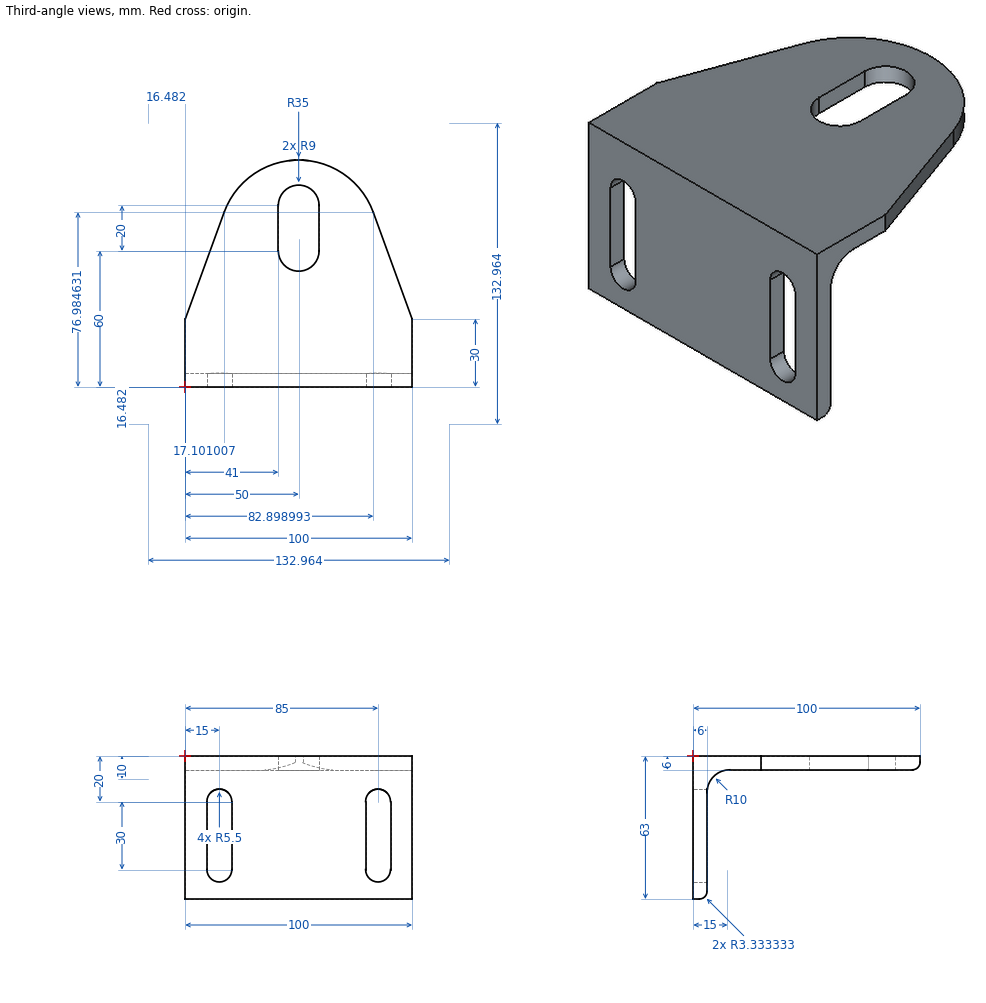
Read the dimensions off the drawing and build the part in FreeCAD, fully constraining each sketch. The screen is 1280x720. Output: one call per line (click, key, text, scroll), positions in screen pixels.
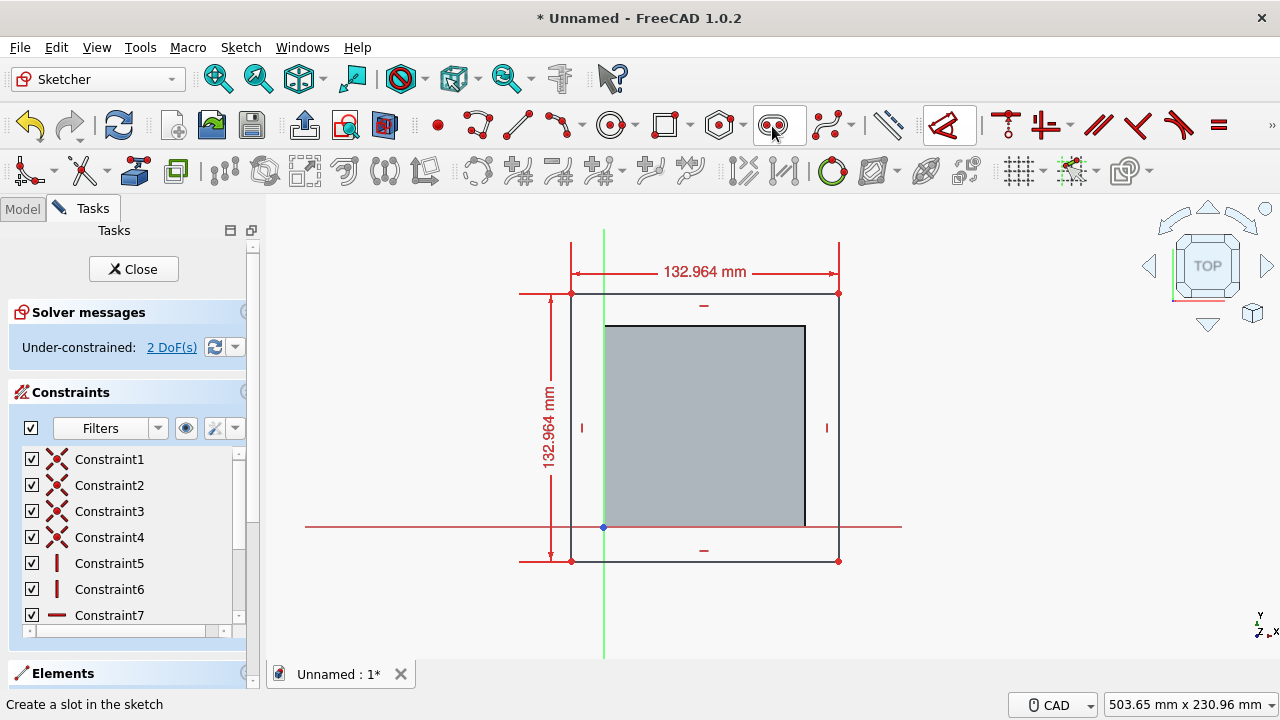
scroll(705, 407, up, 2)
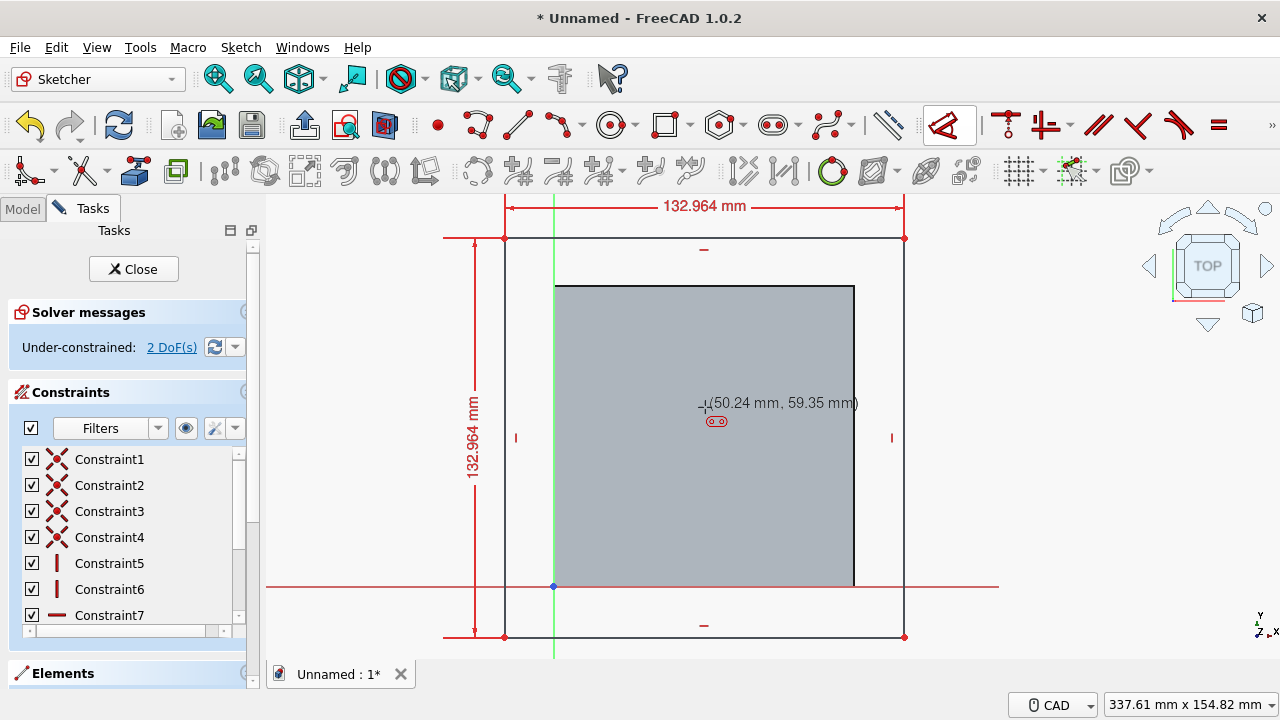
click(704, 406)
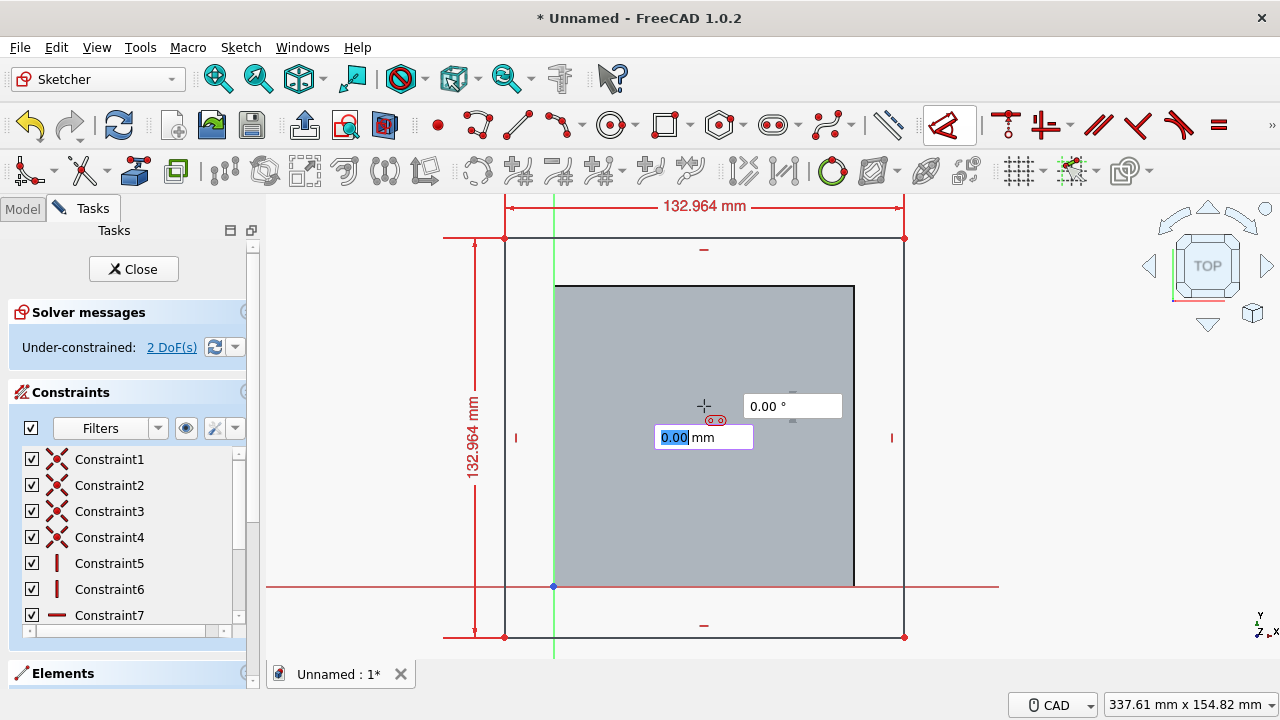
click(704, 346)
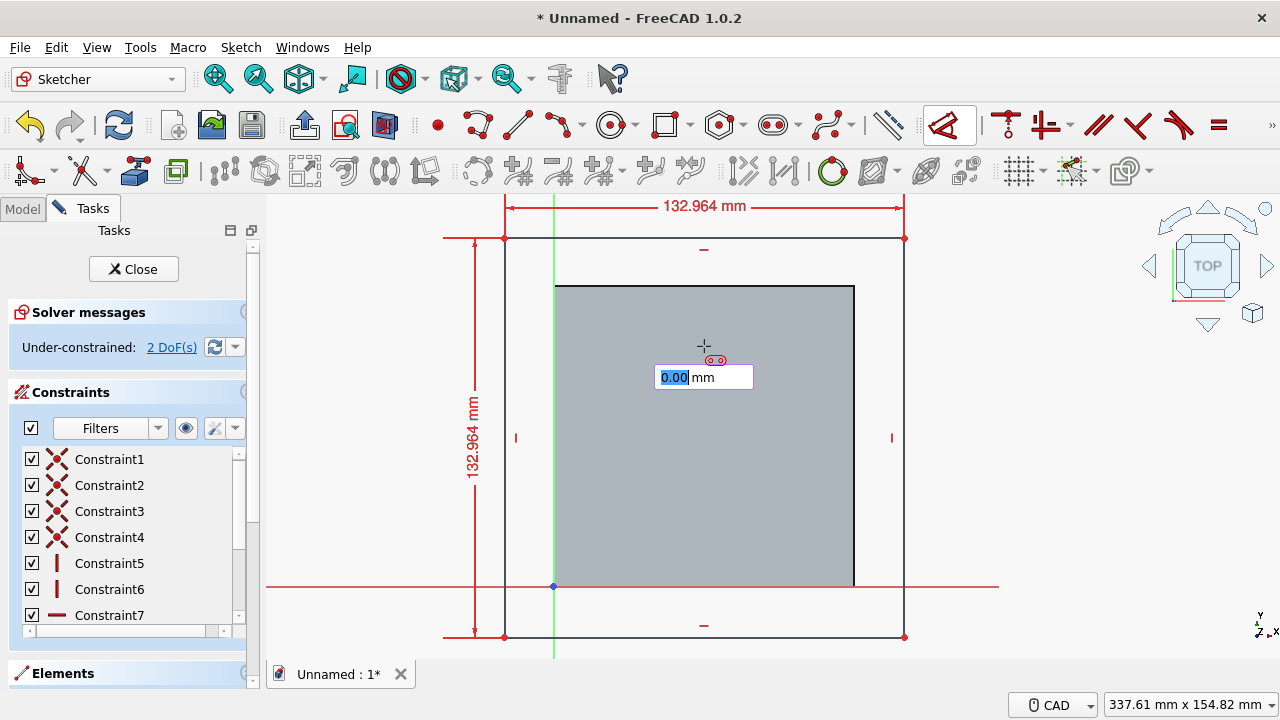
click(731, 376)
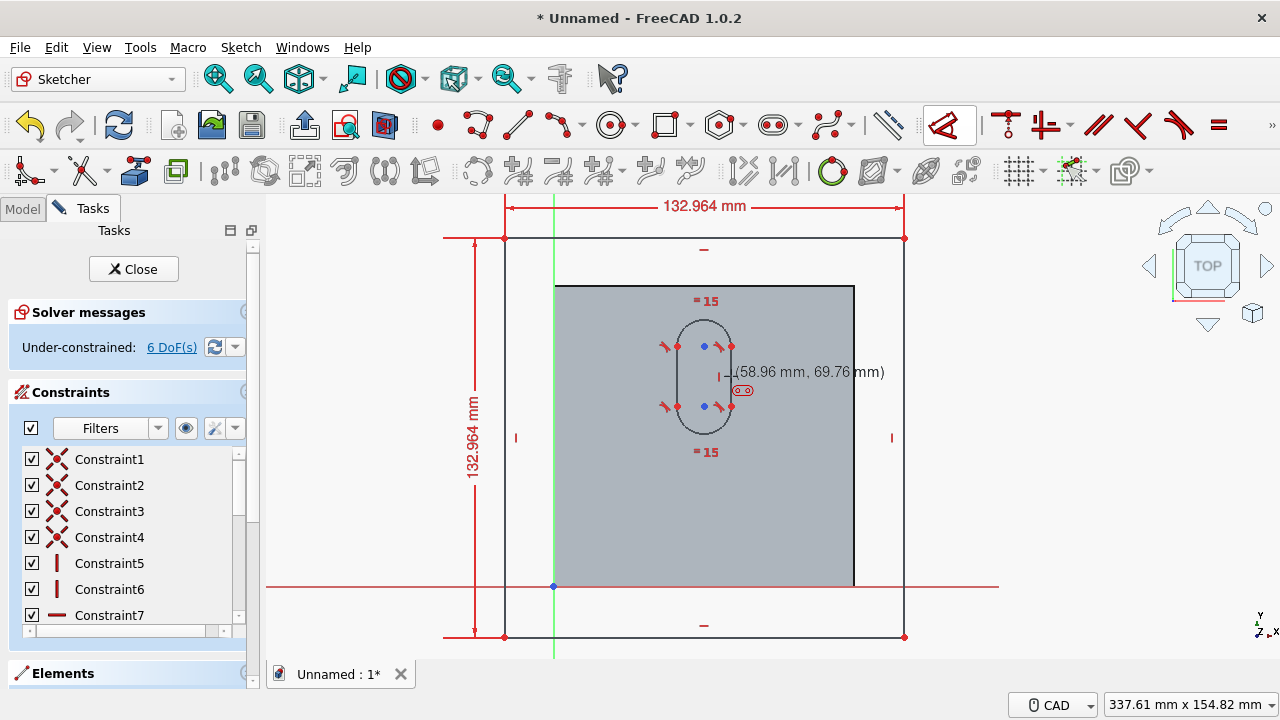
click(478, 126)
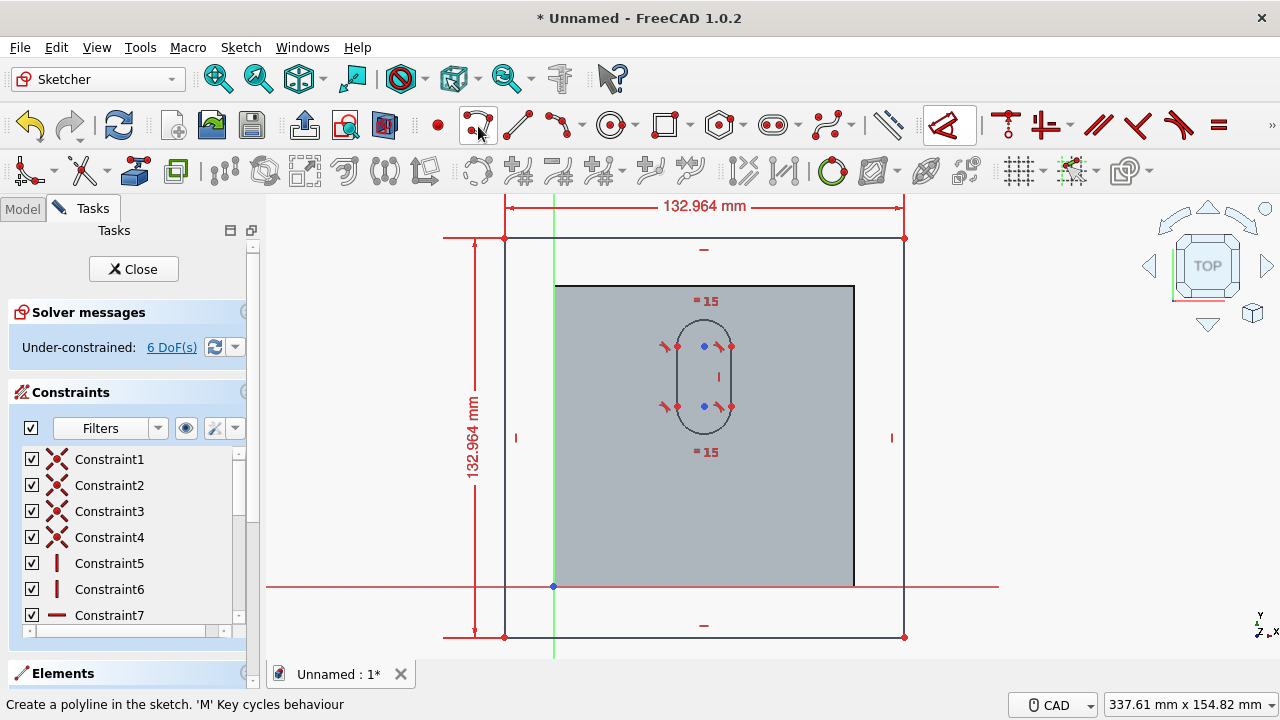
click(803, 355)
click(854, 496)
click(854, 587)
click(554, 587)
click(563, 496)
click(605, 355)
right_click(605, 355)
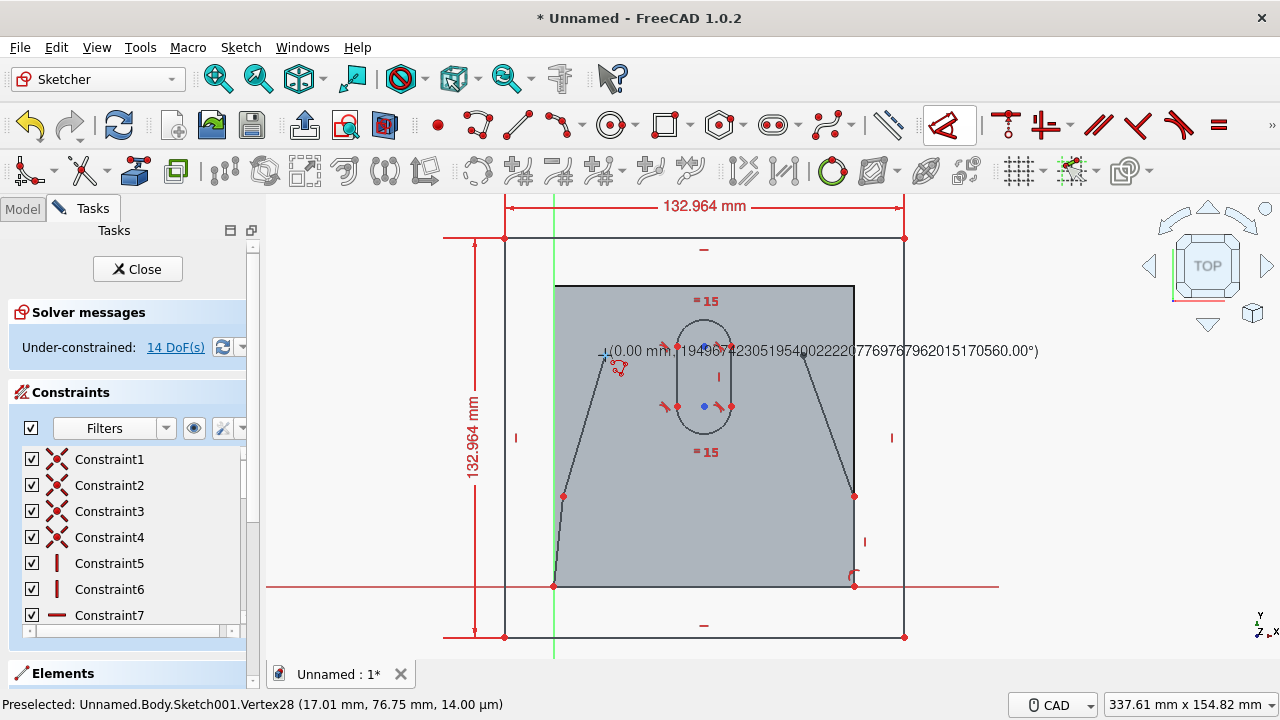
click(558, 126)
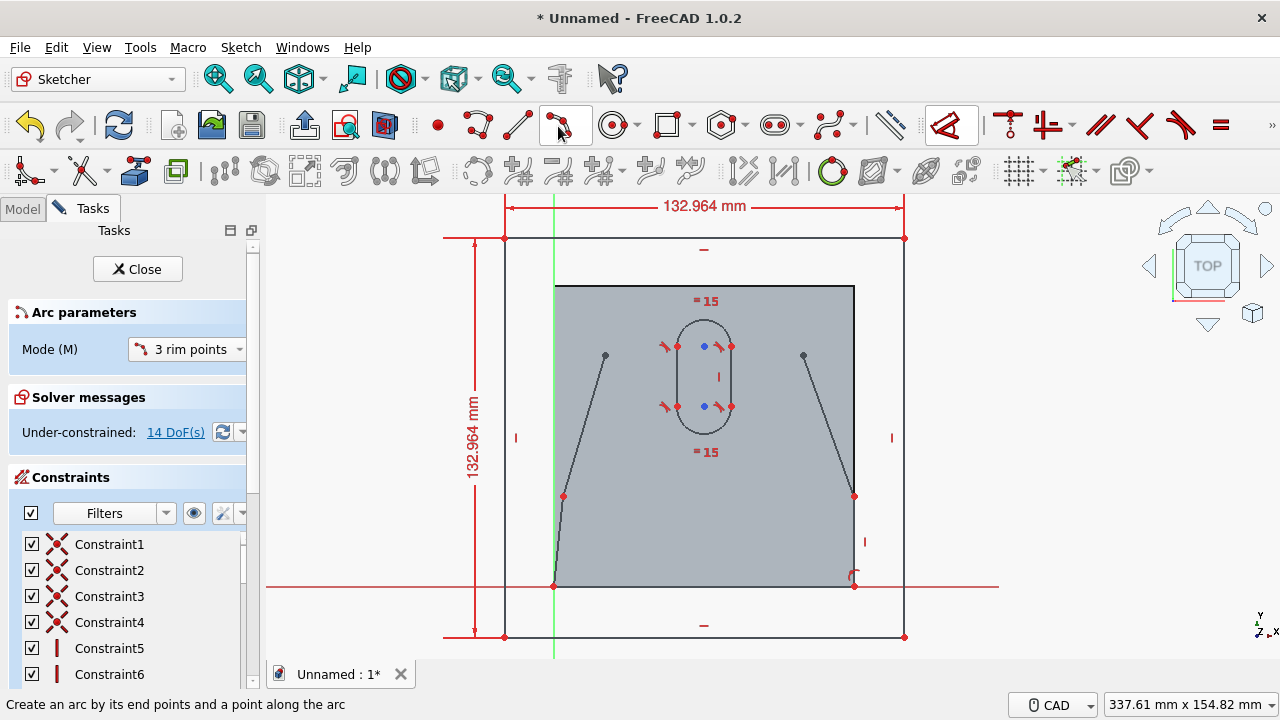
click(605, 356)
click(803, 356)
click(704, 286)
key(Escape)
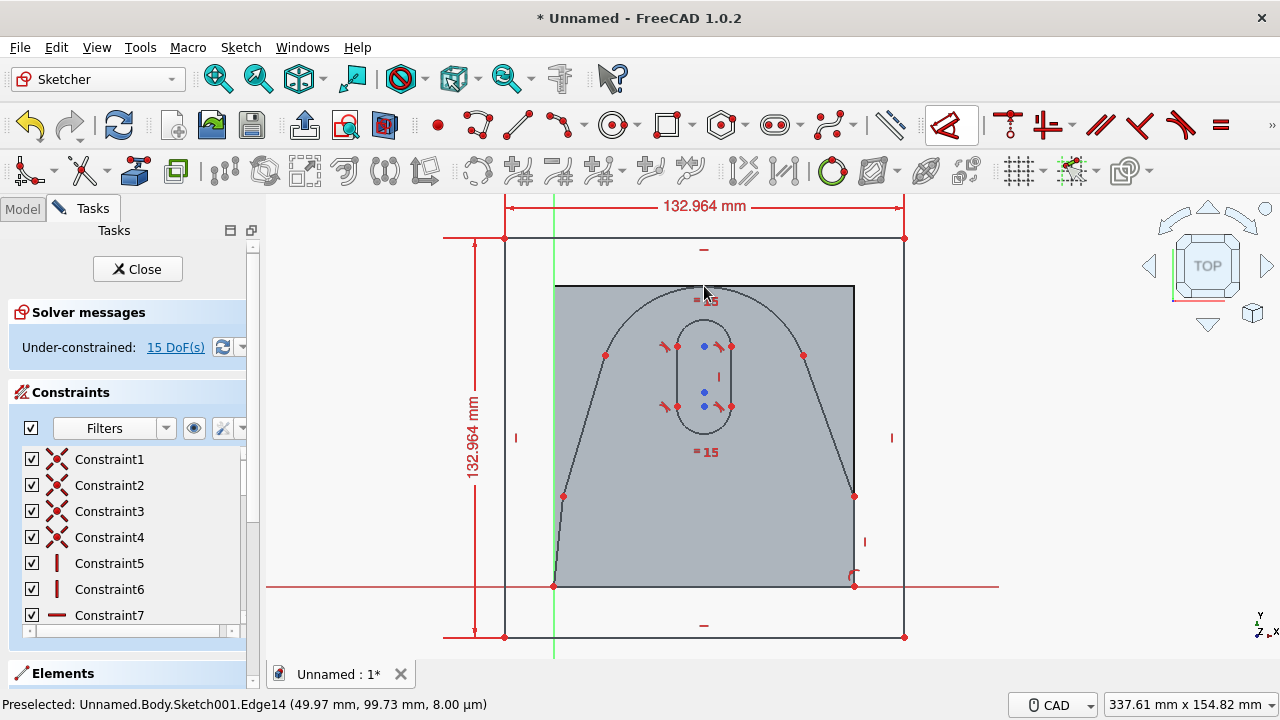
click(557, 560)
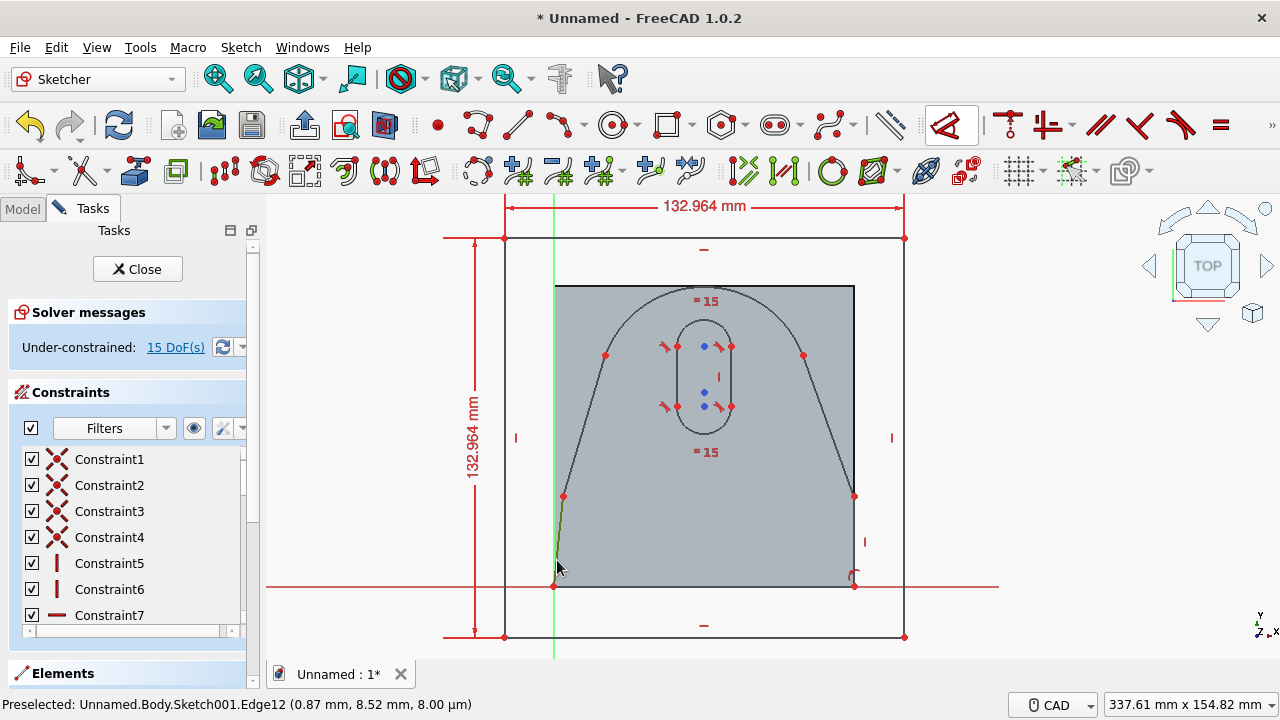
key(v)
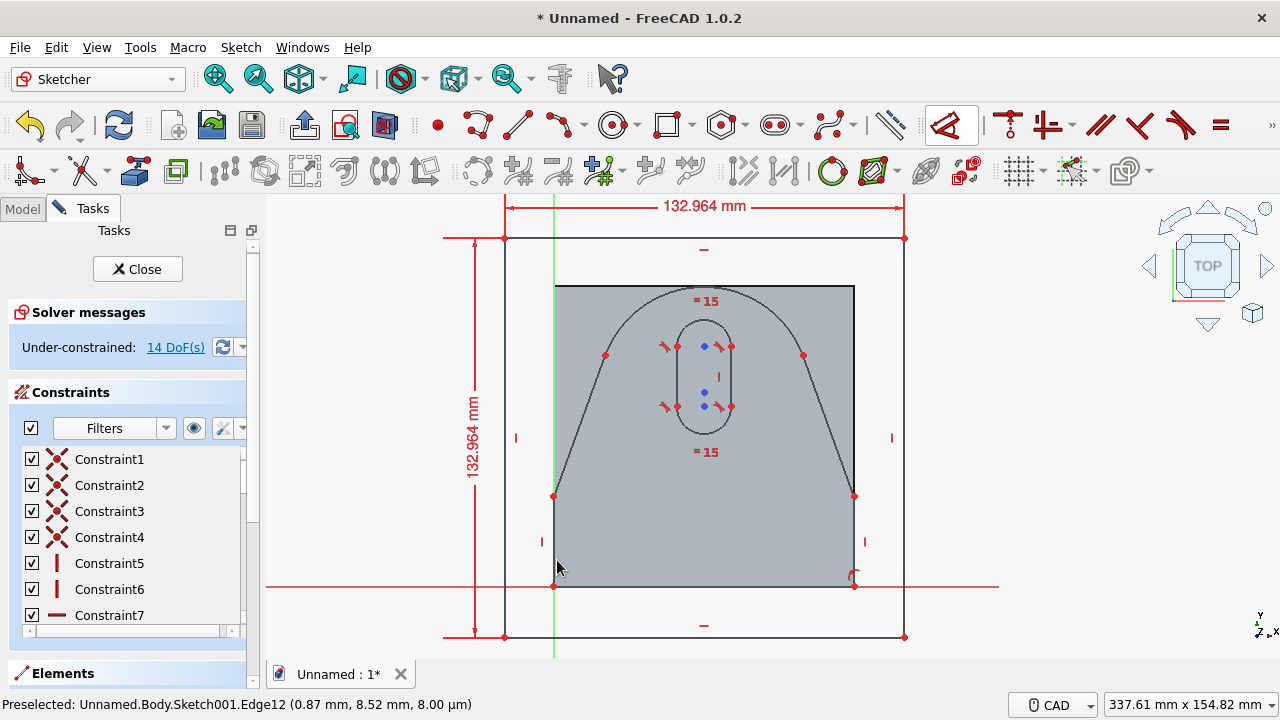
scroll(688, 429, up, 2)